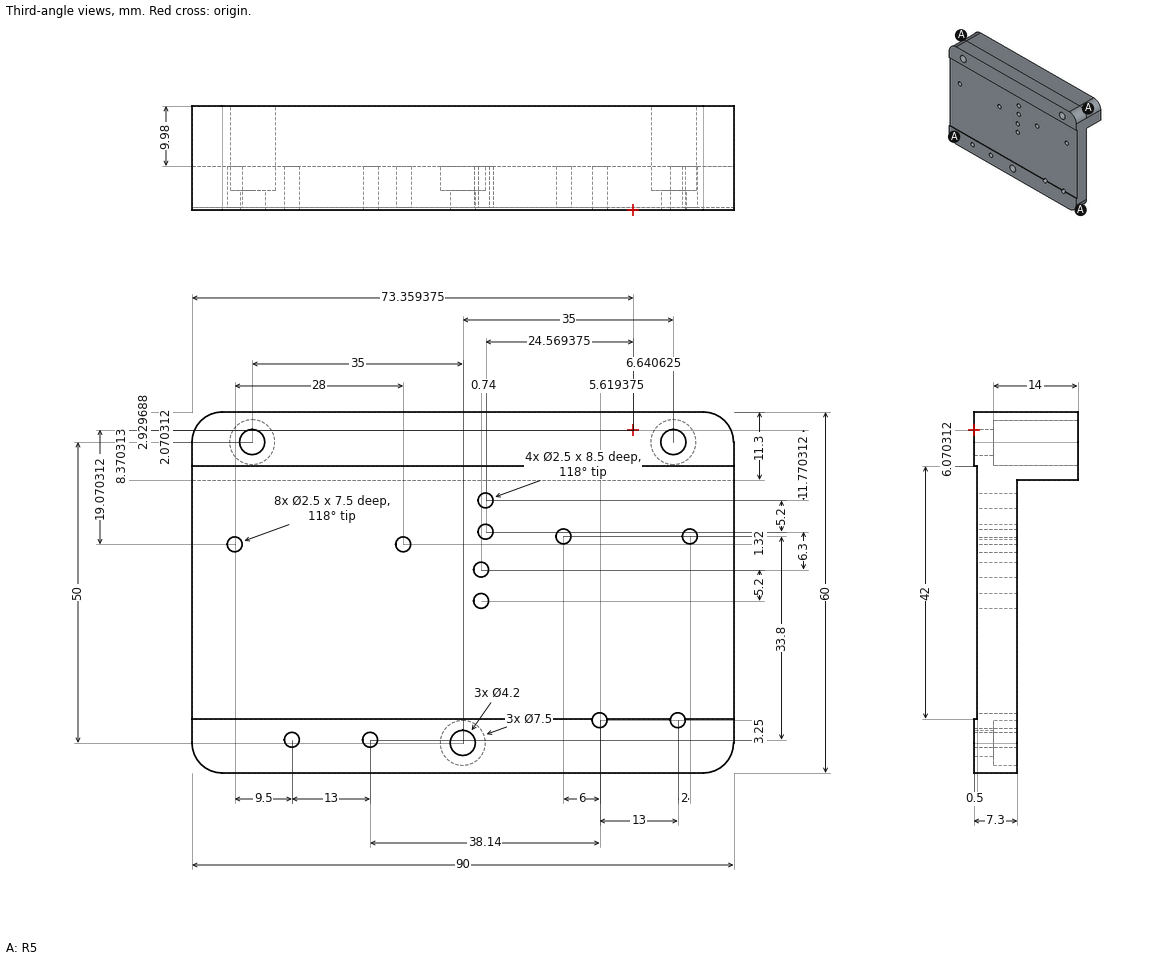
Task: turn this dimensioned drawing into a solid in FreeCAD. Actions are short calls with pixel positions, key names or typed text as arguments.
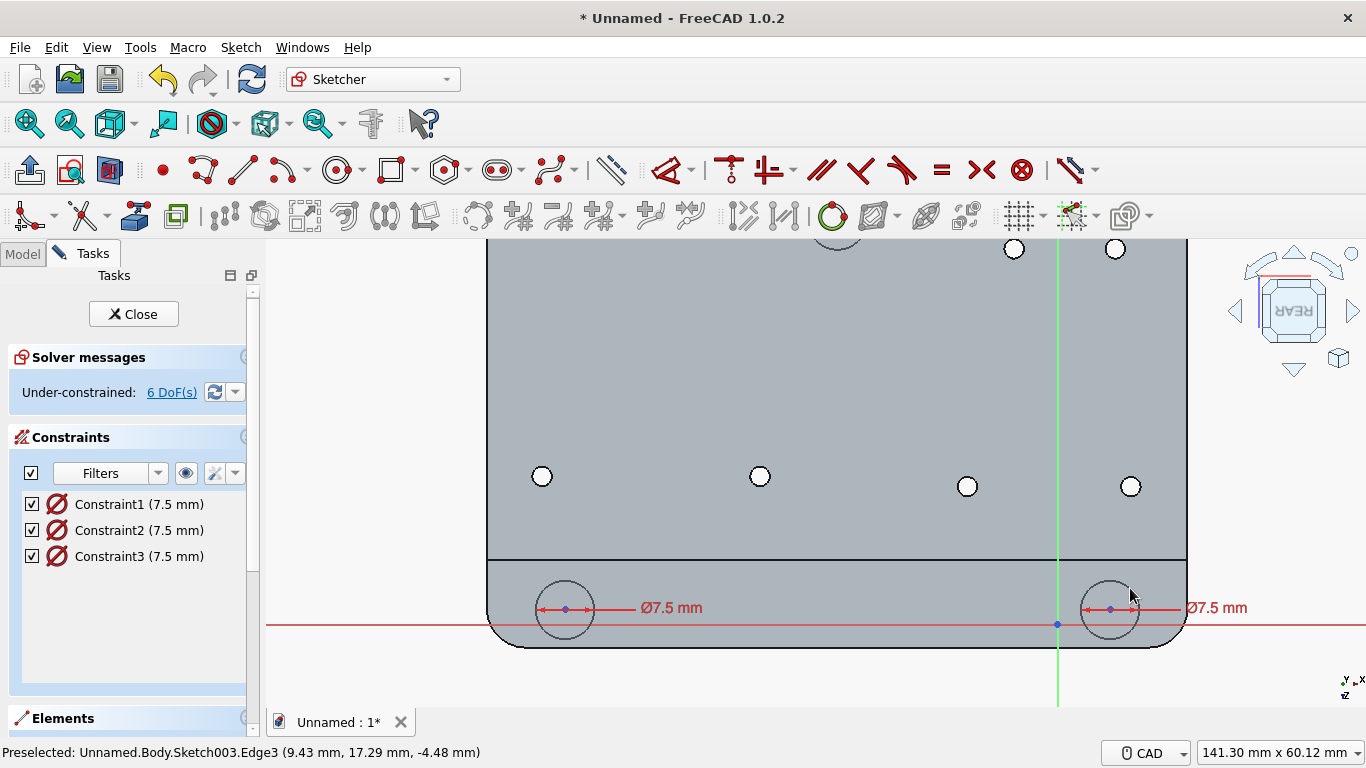
click(666, 170)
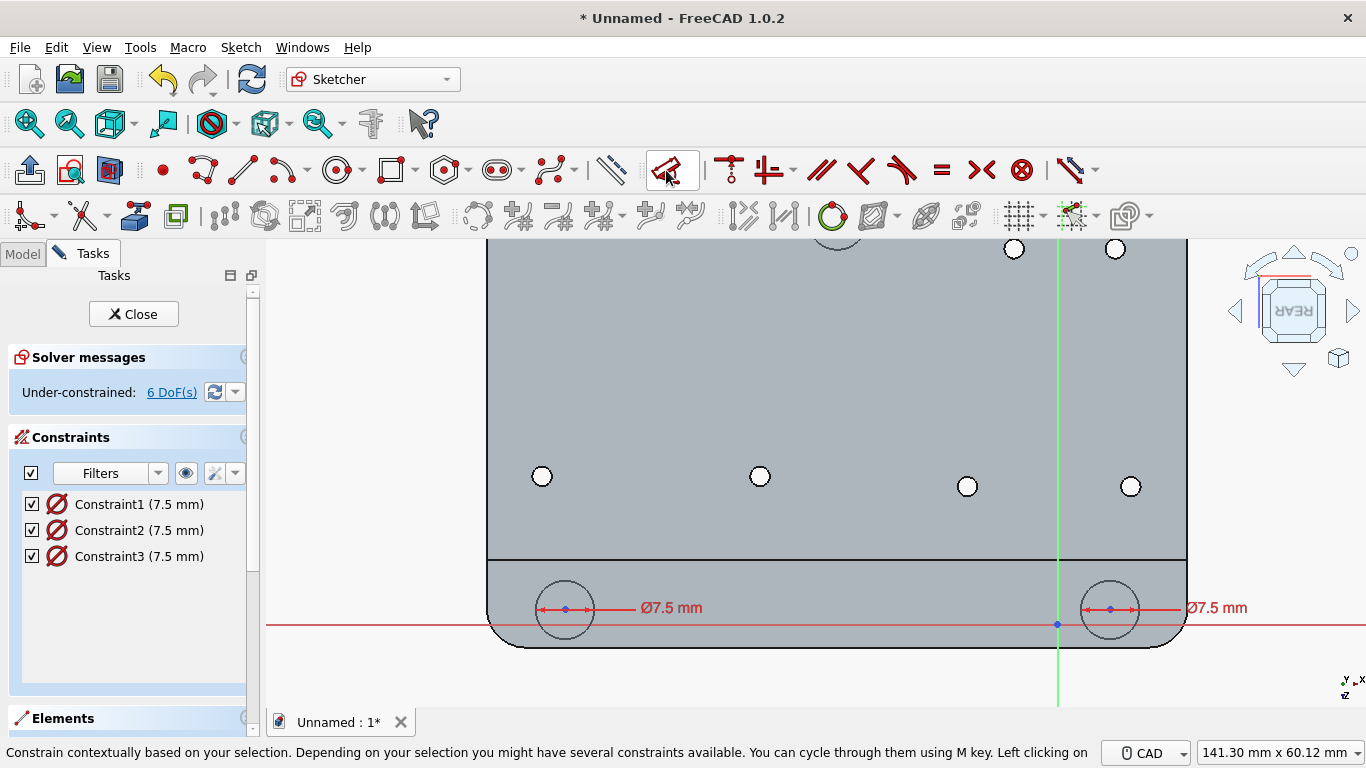
scroll(565, 593, down, 2)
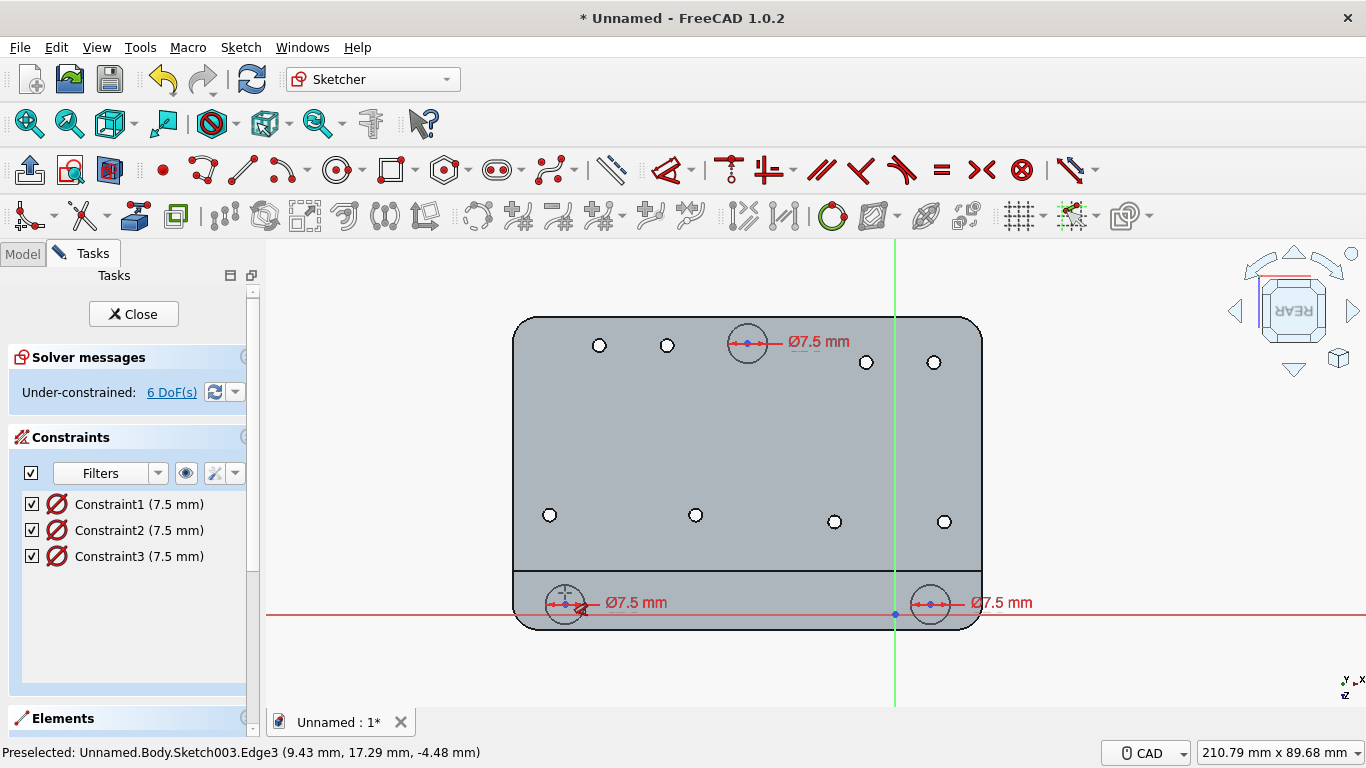
click(748, 344)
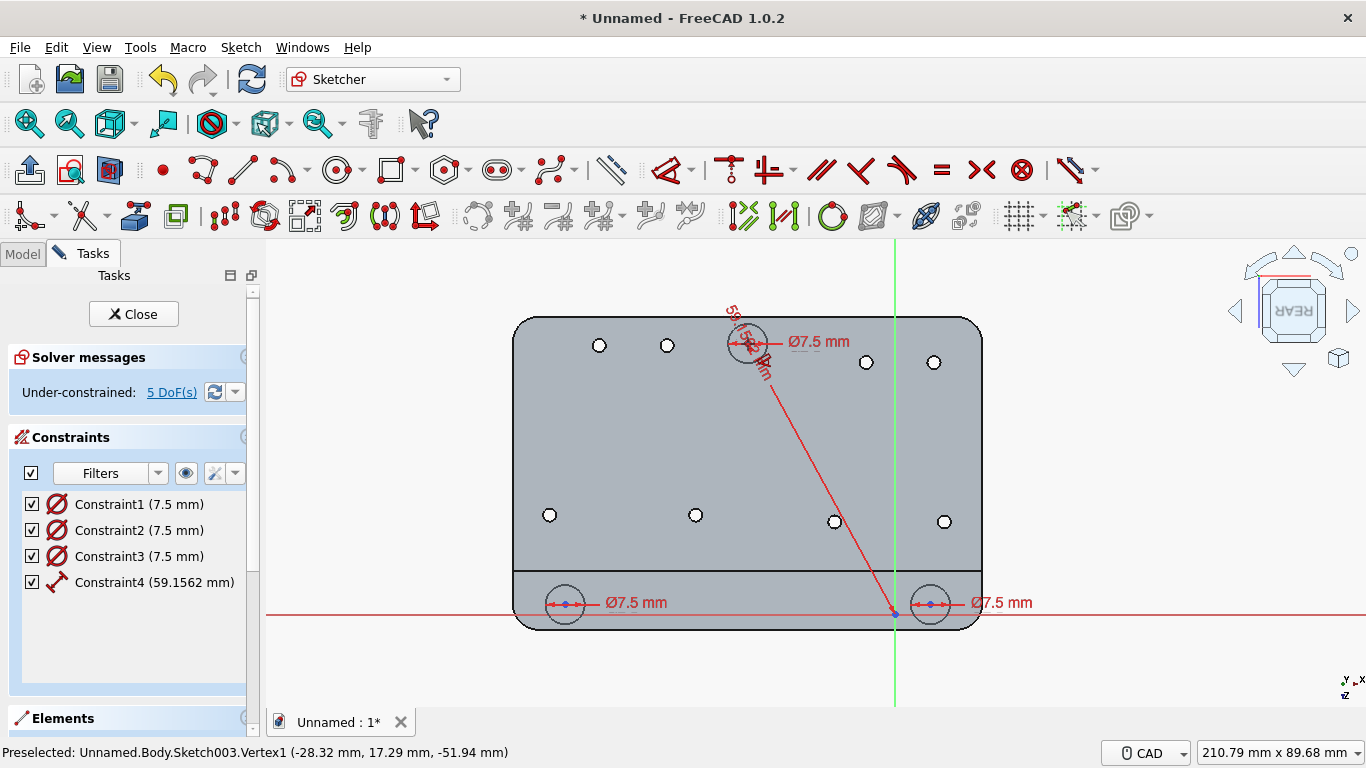
click(565, 605)
click(656, 639)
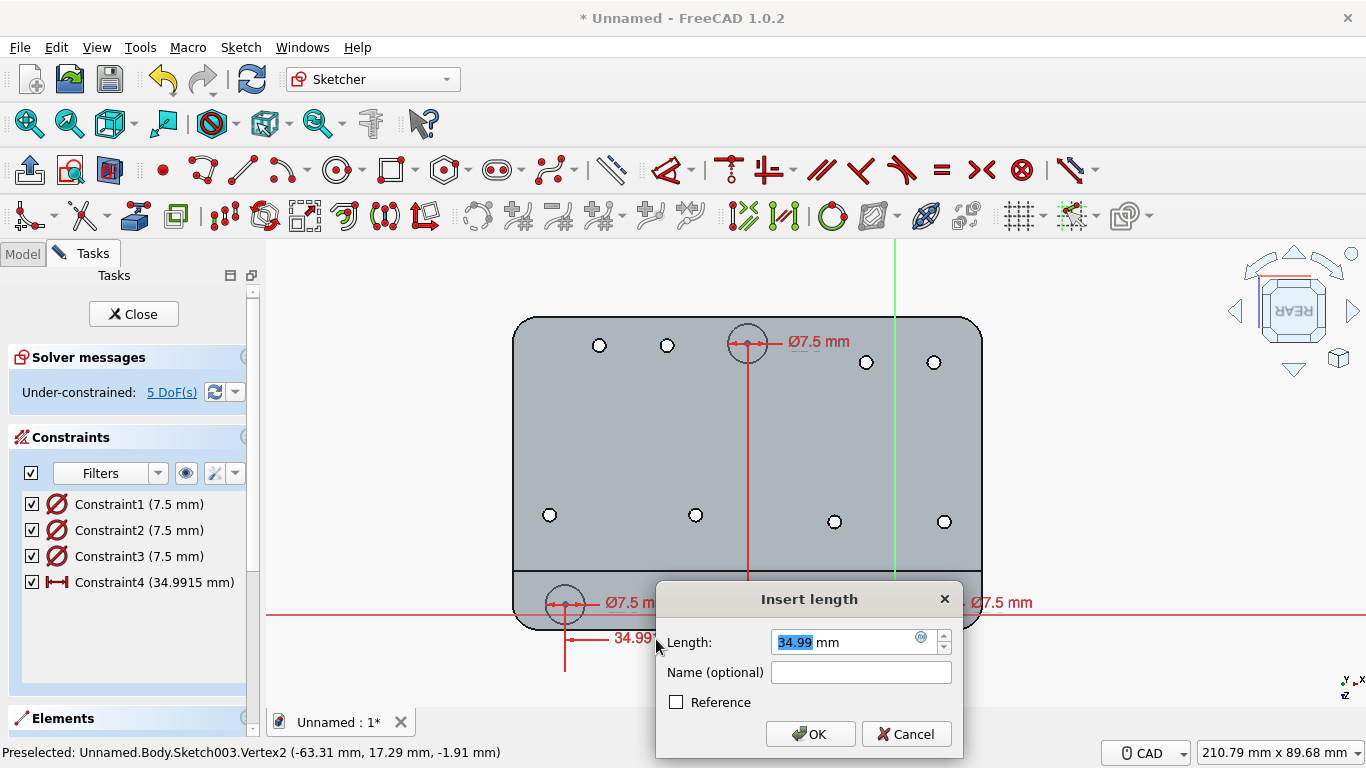
text(35)
key(Return)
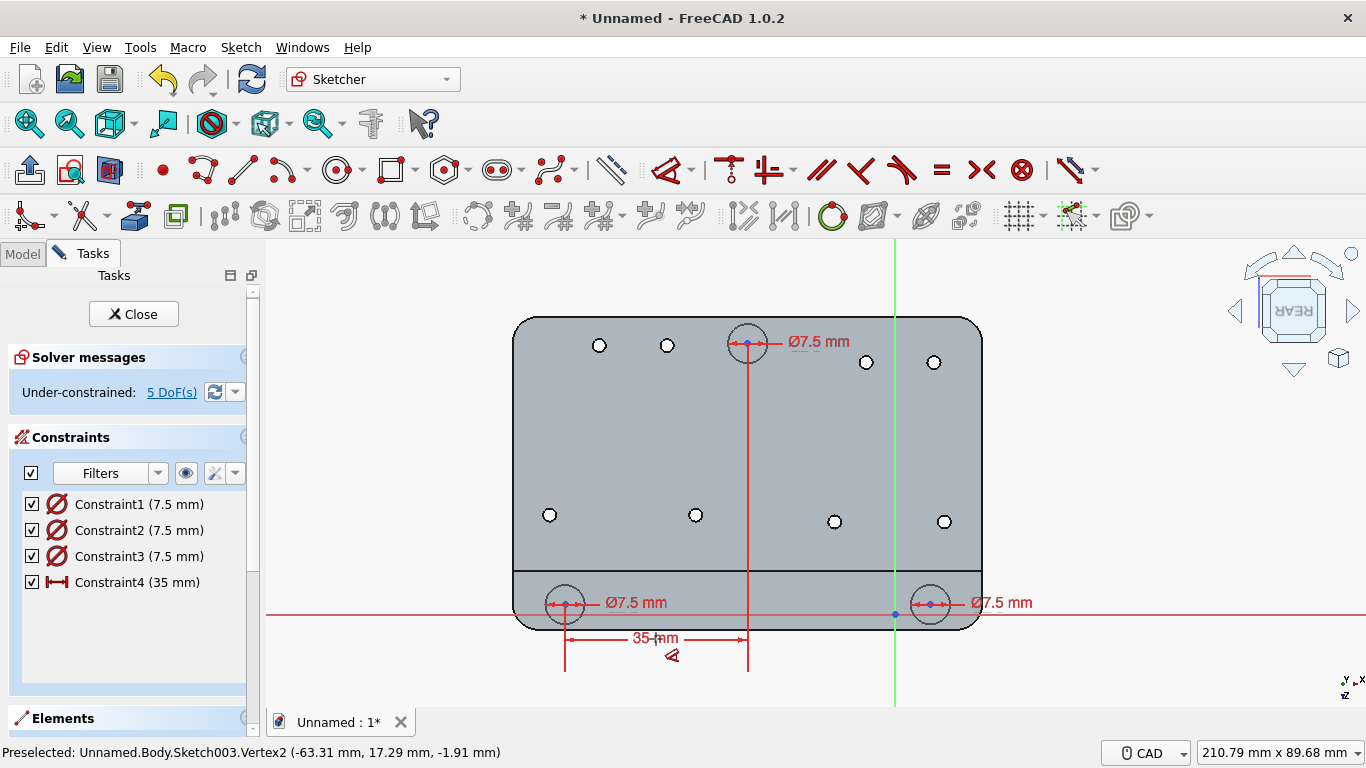
click(748, 344)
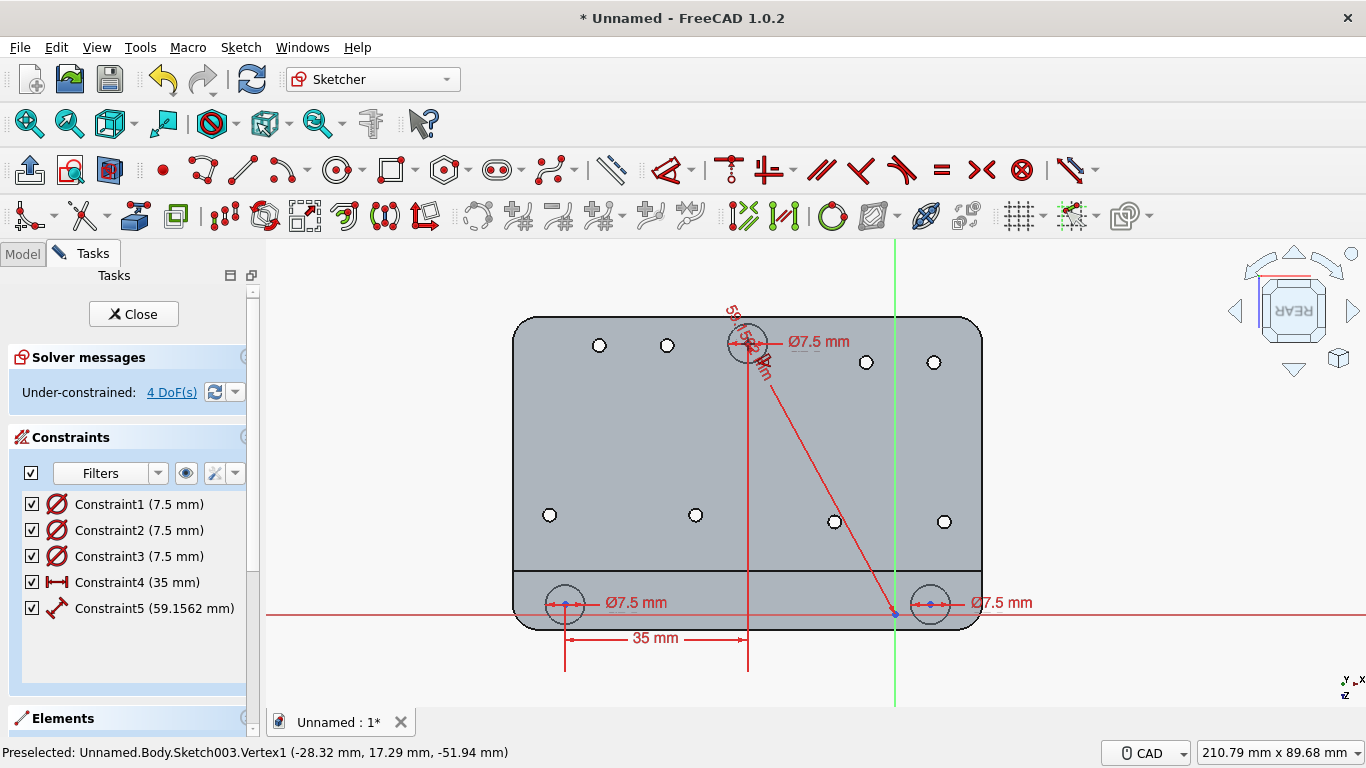
click(565, 605)
click(531, 474)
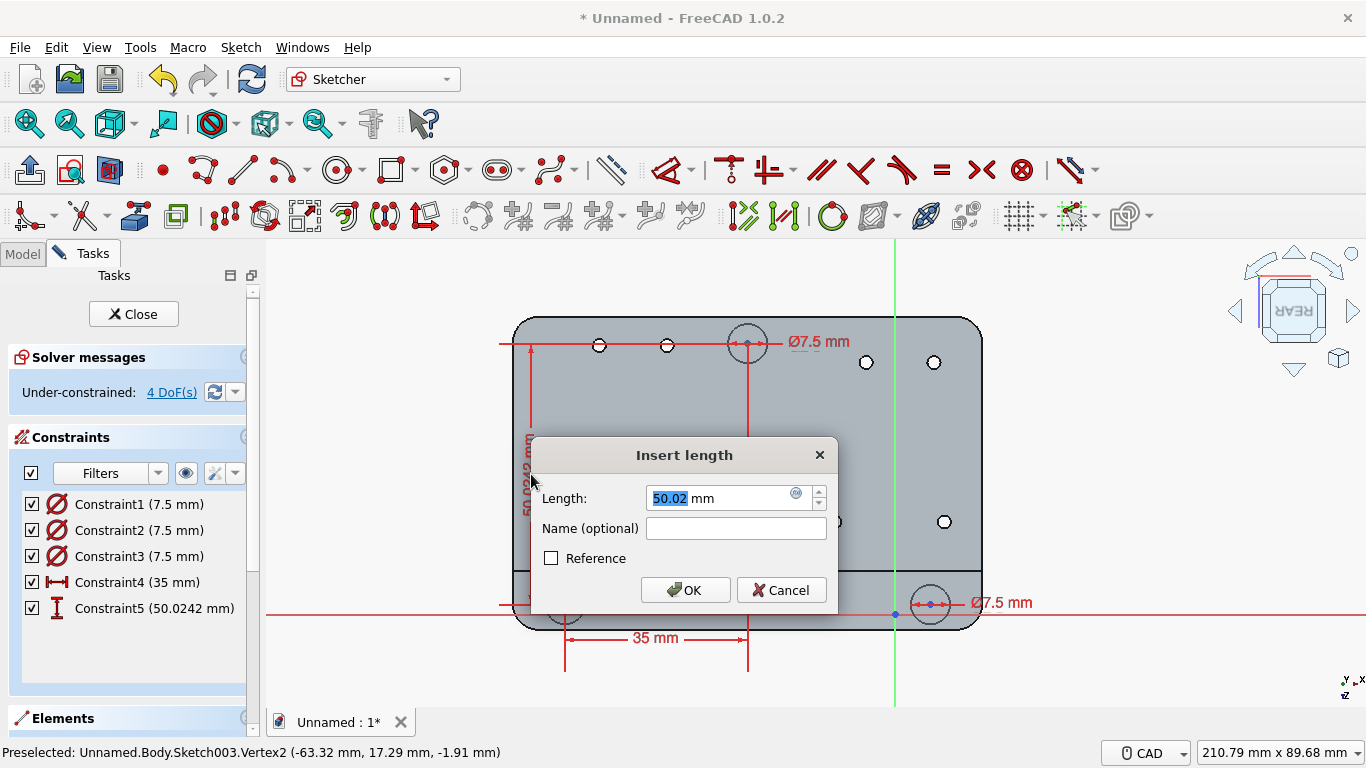
text(50)
key(Return)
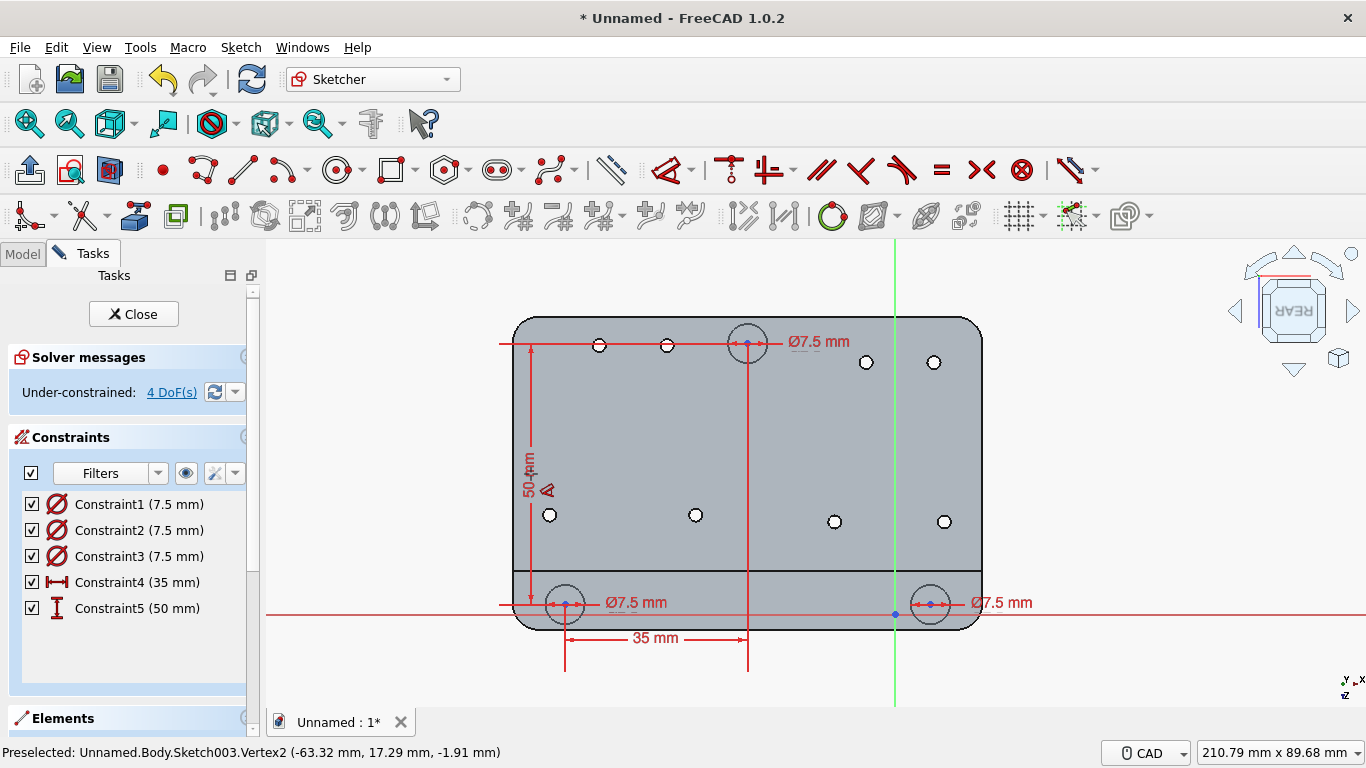
click(748, 344)